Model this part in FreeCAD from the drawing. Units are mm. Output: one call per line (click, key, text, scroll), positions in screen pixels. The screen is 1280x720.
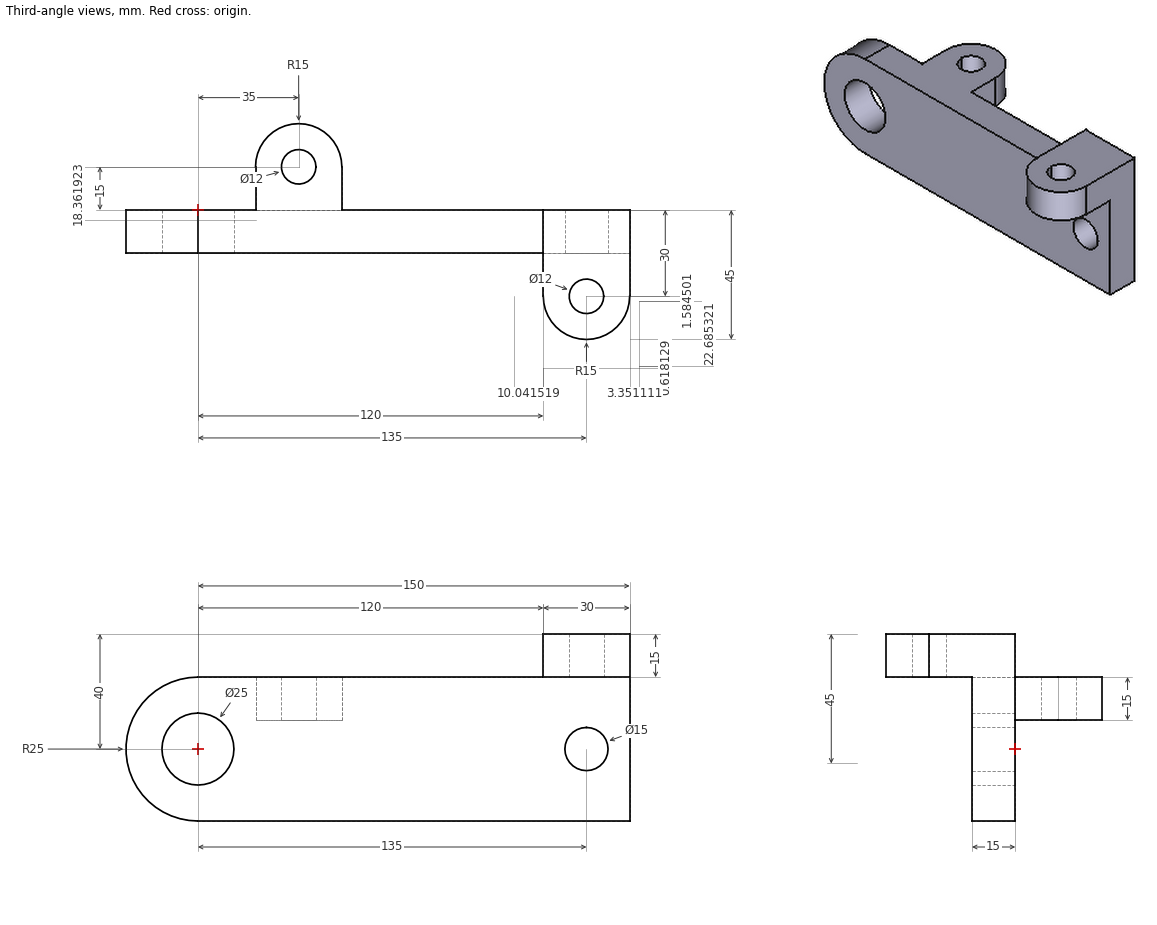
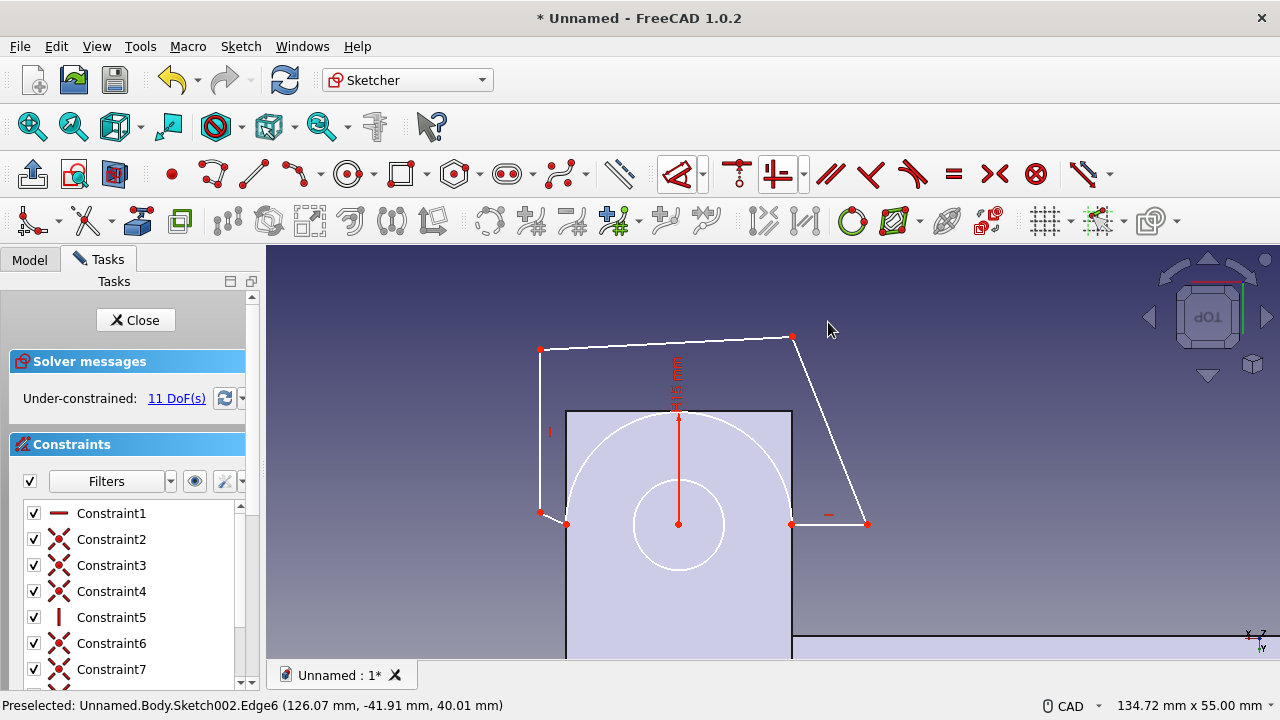
click(711, 493)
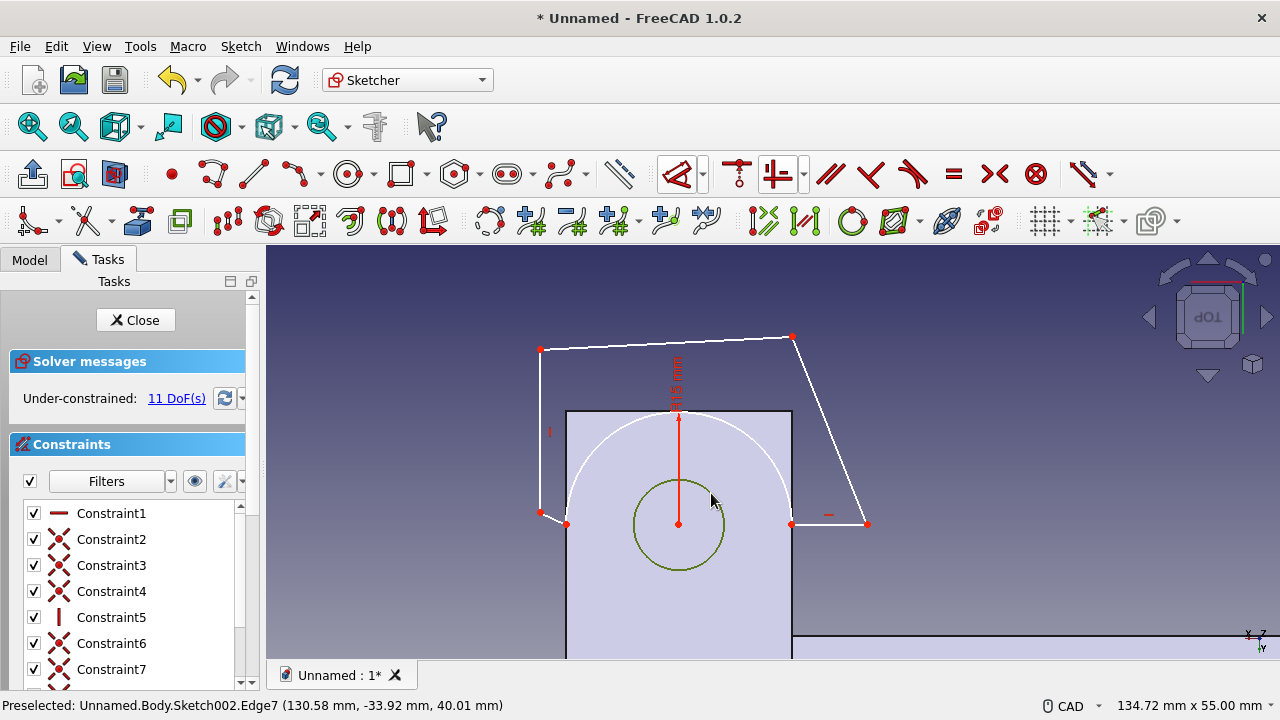
key(k)
key(o)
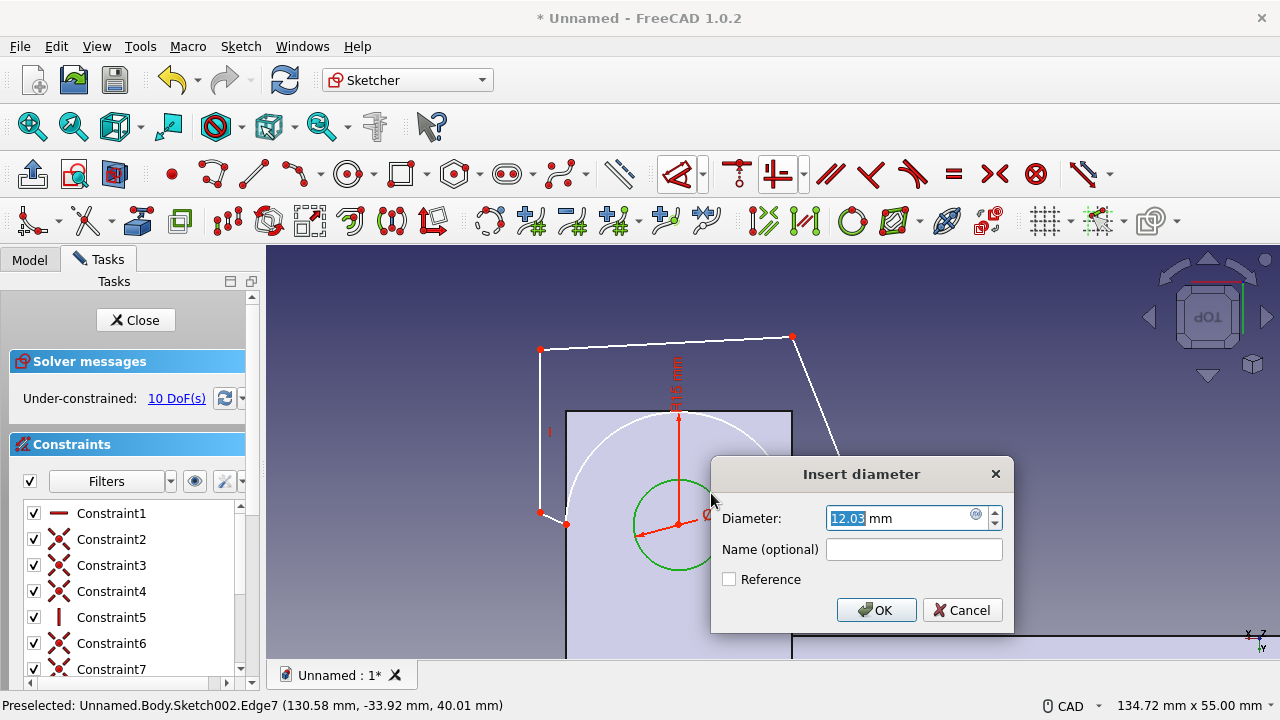
text(12)
key(Return)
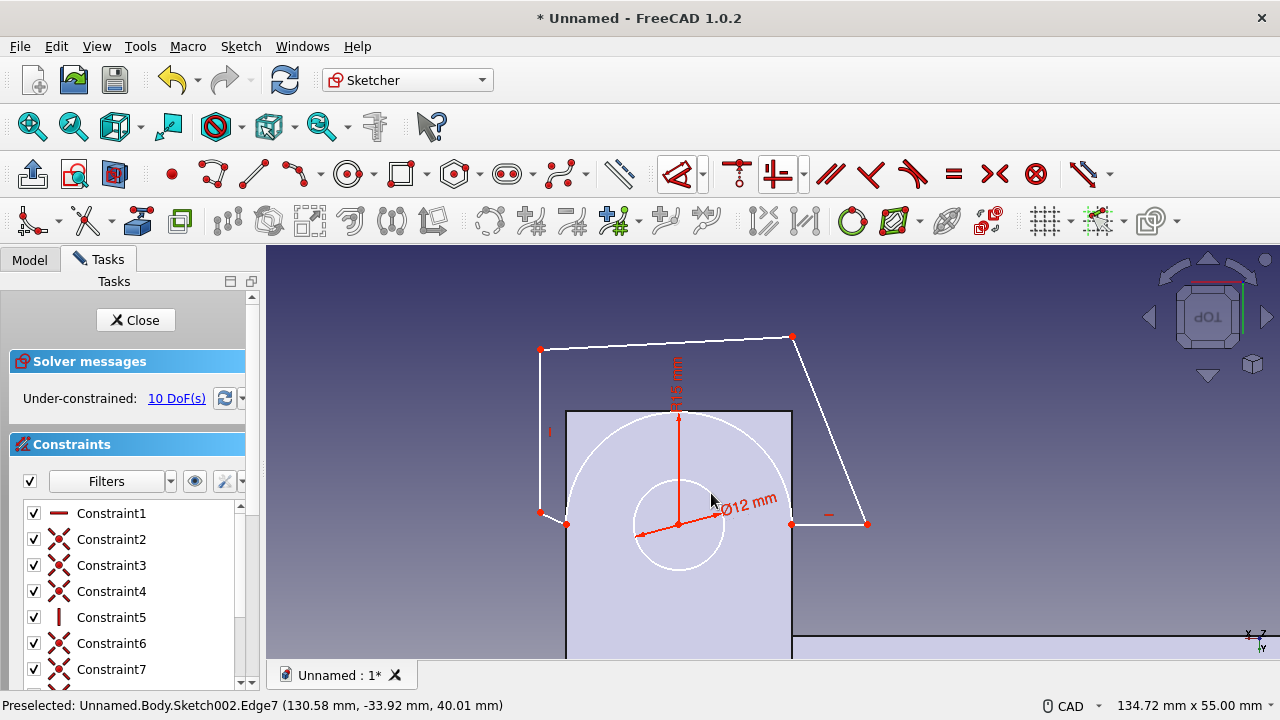
click(679, 525)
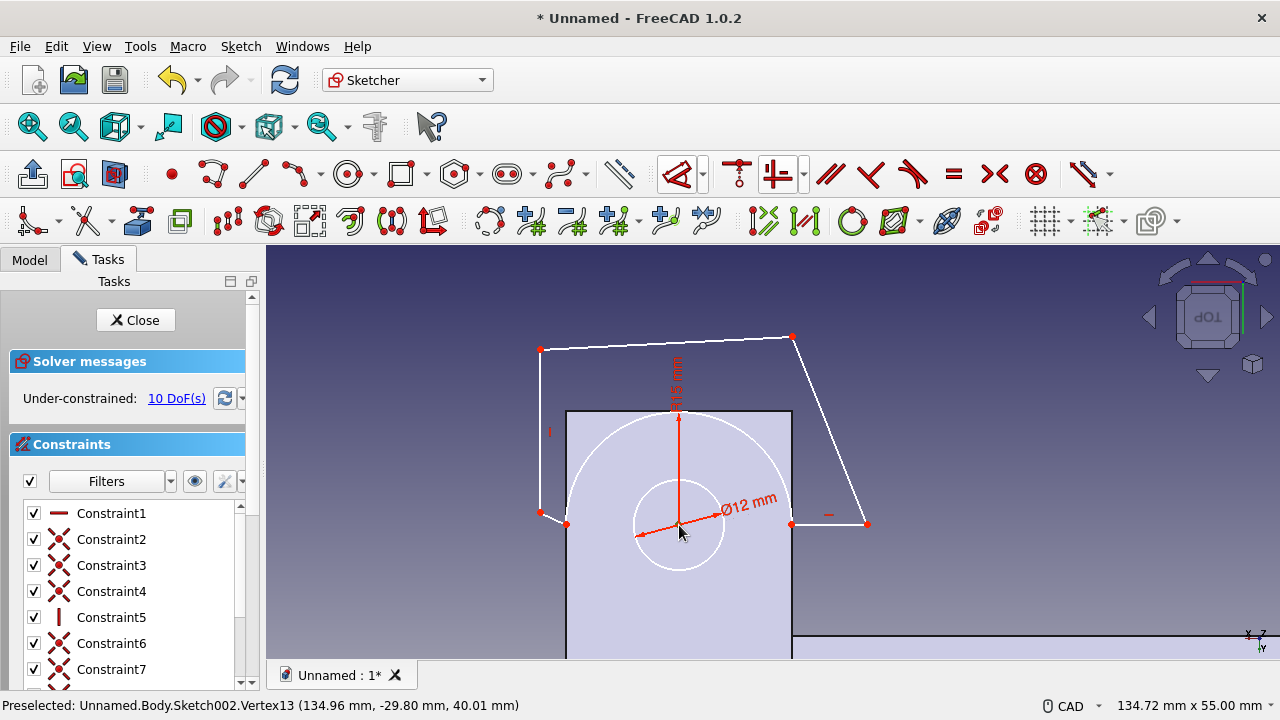
key(i)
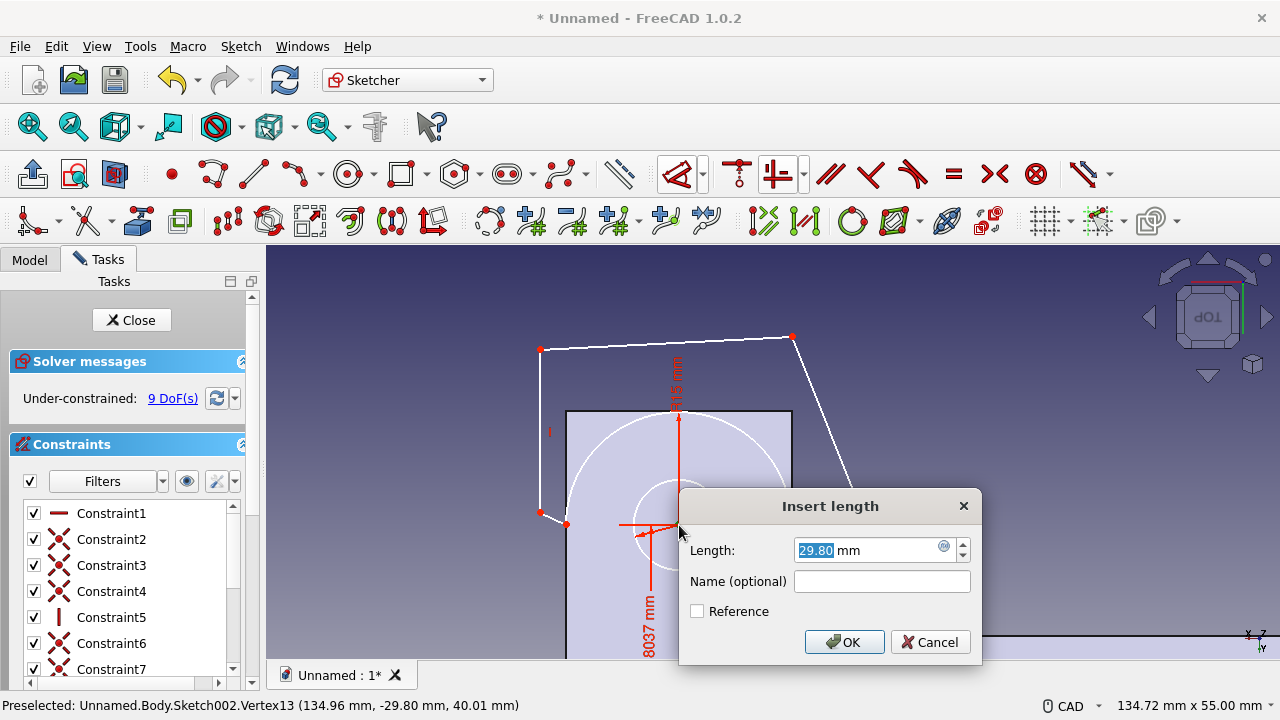
text(30)
key(Return)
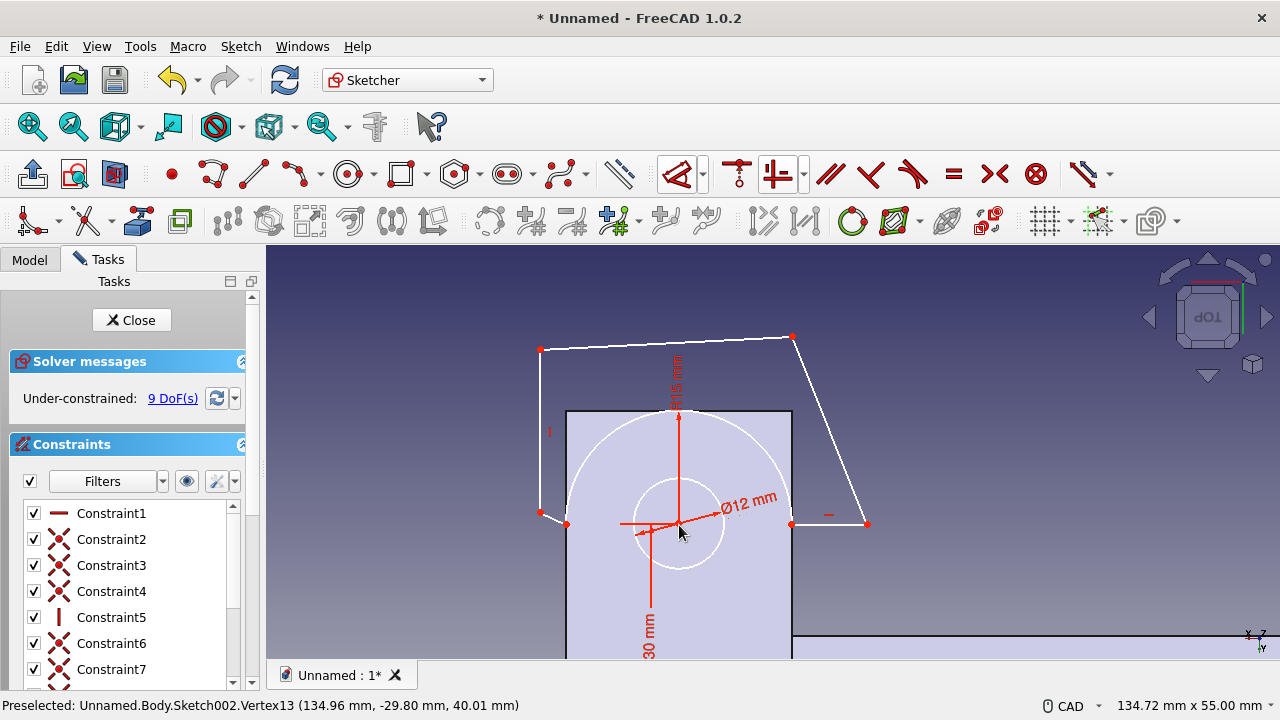
click(792, 525)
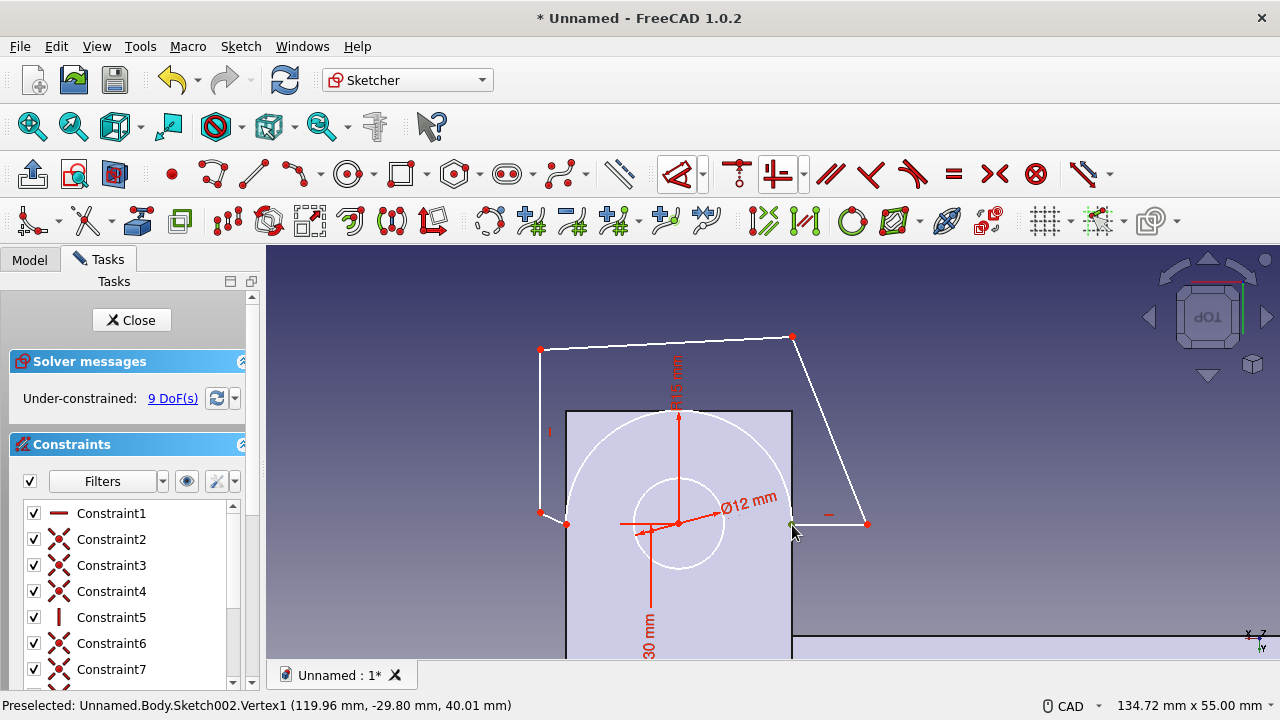
click(702, 174)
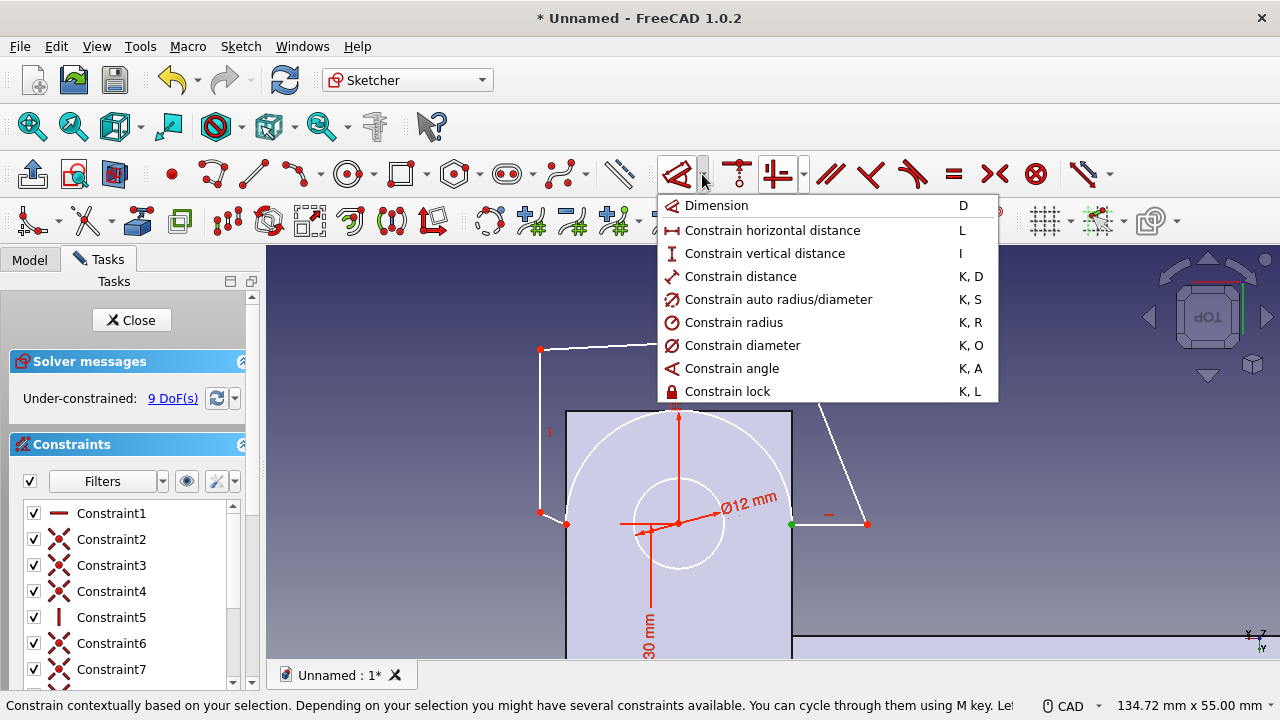
click(828, 254)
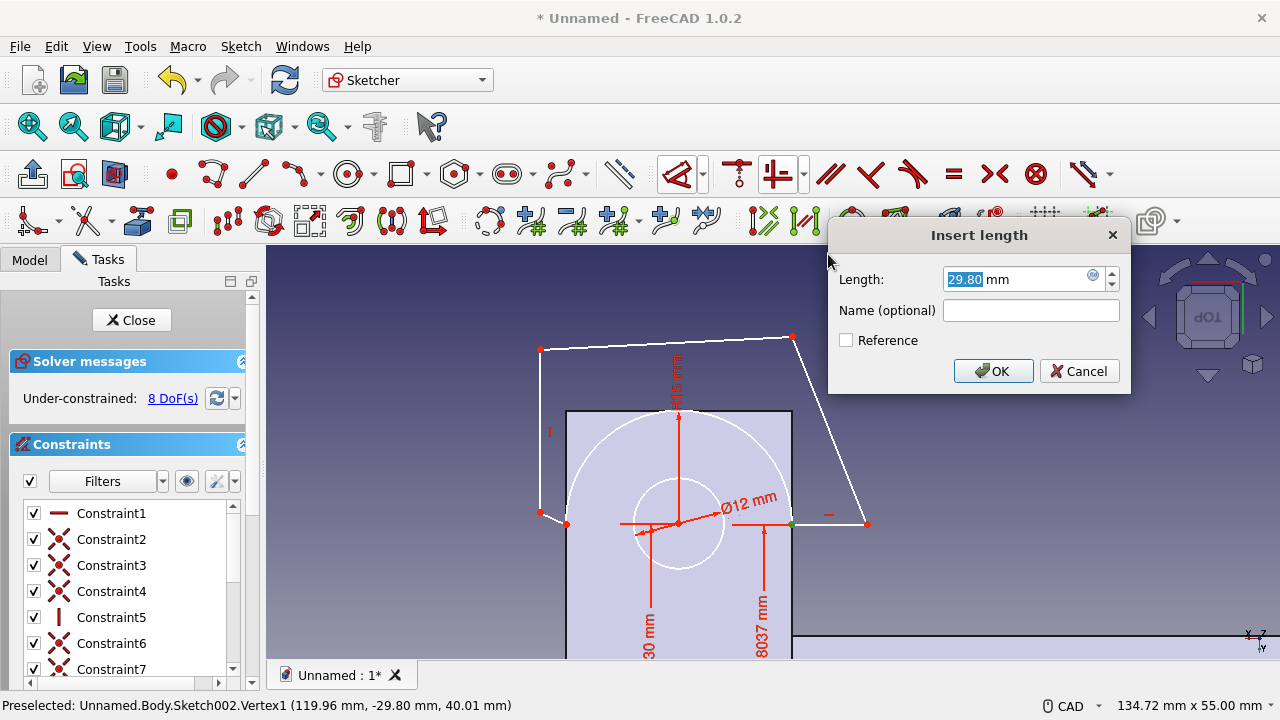
text(30)
key(Return)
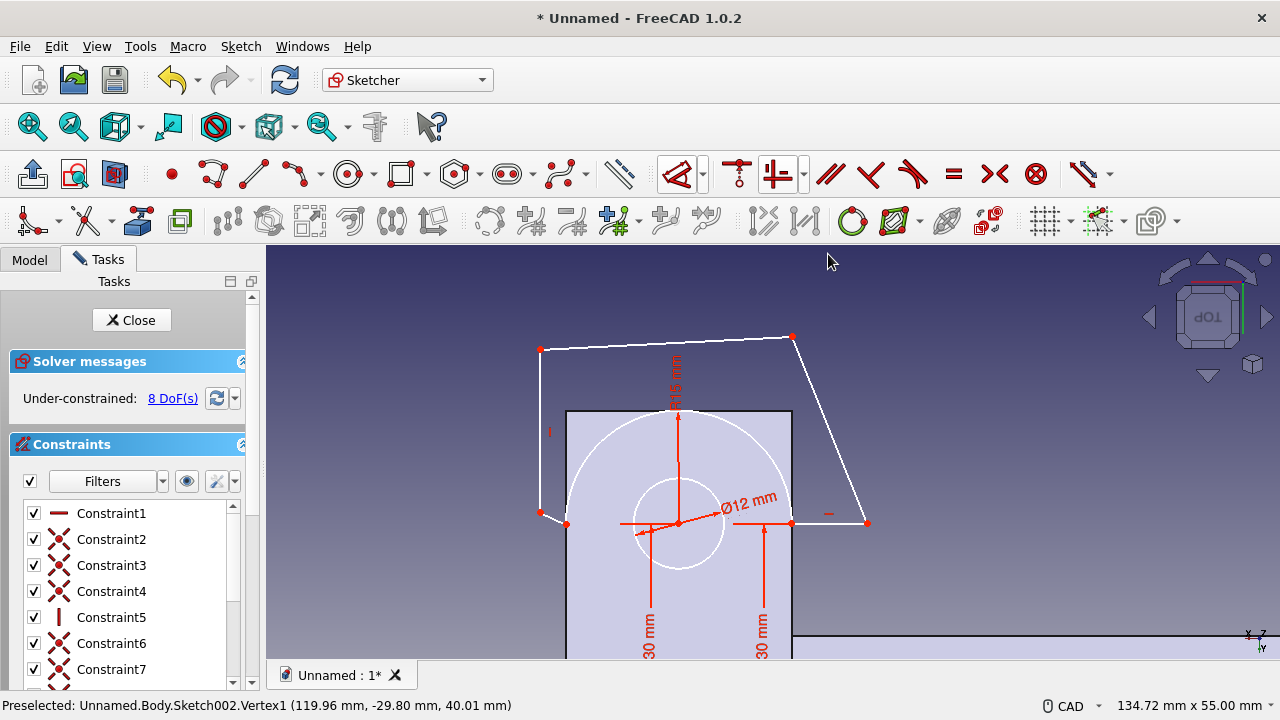
click(566, 525)